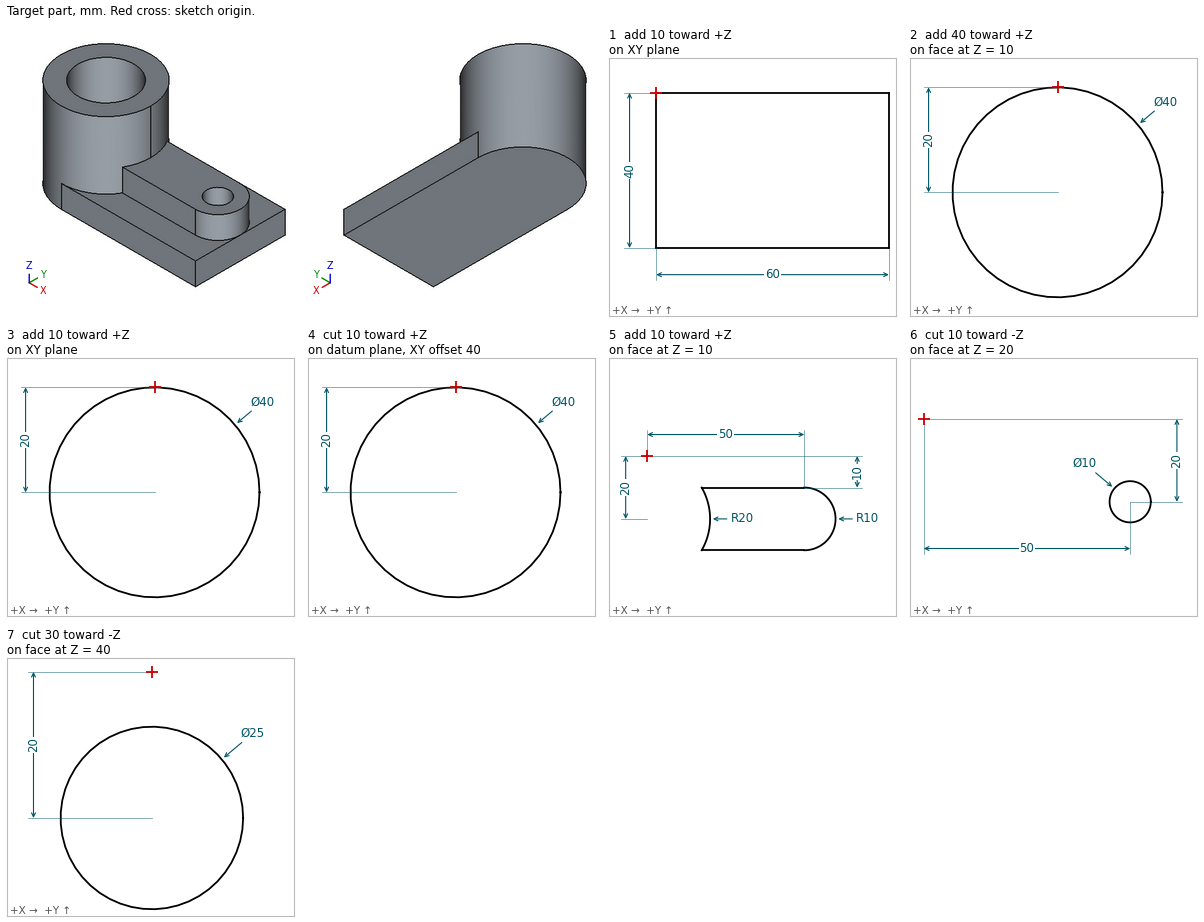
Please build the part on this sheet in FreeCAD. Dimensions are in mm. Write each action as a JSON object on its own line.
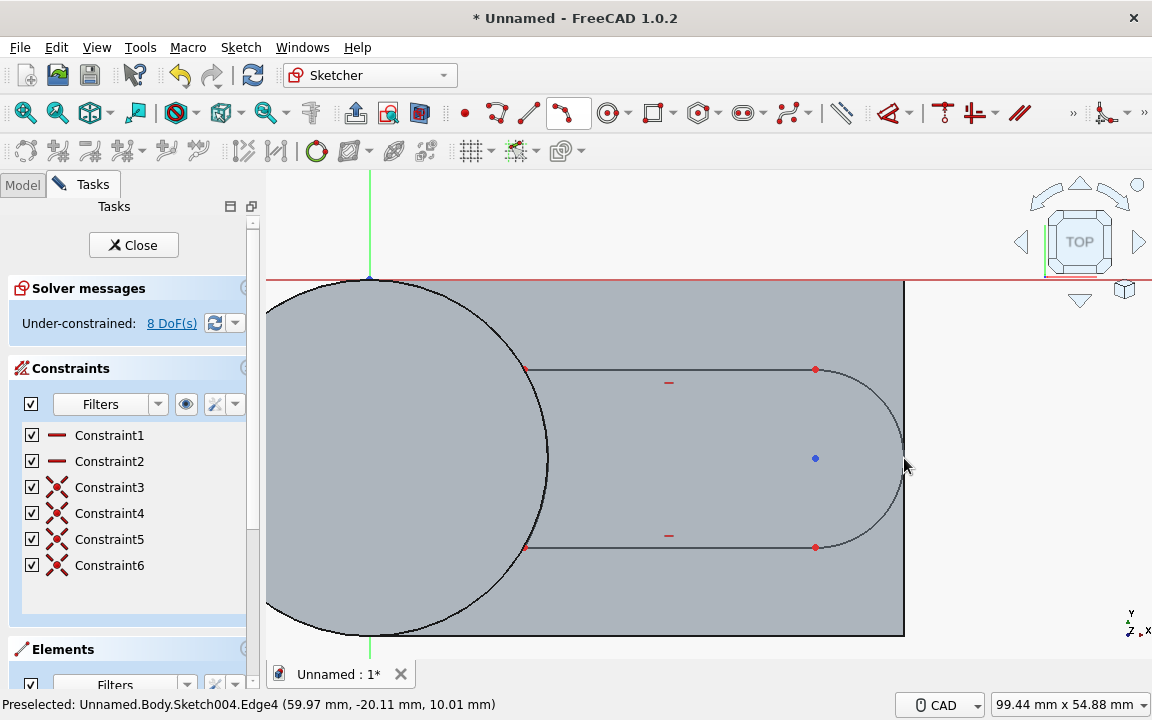
{"action": "left_click", "coordinate": [728, 370]}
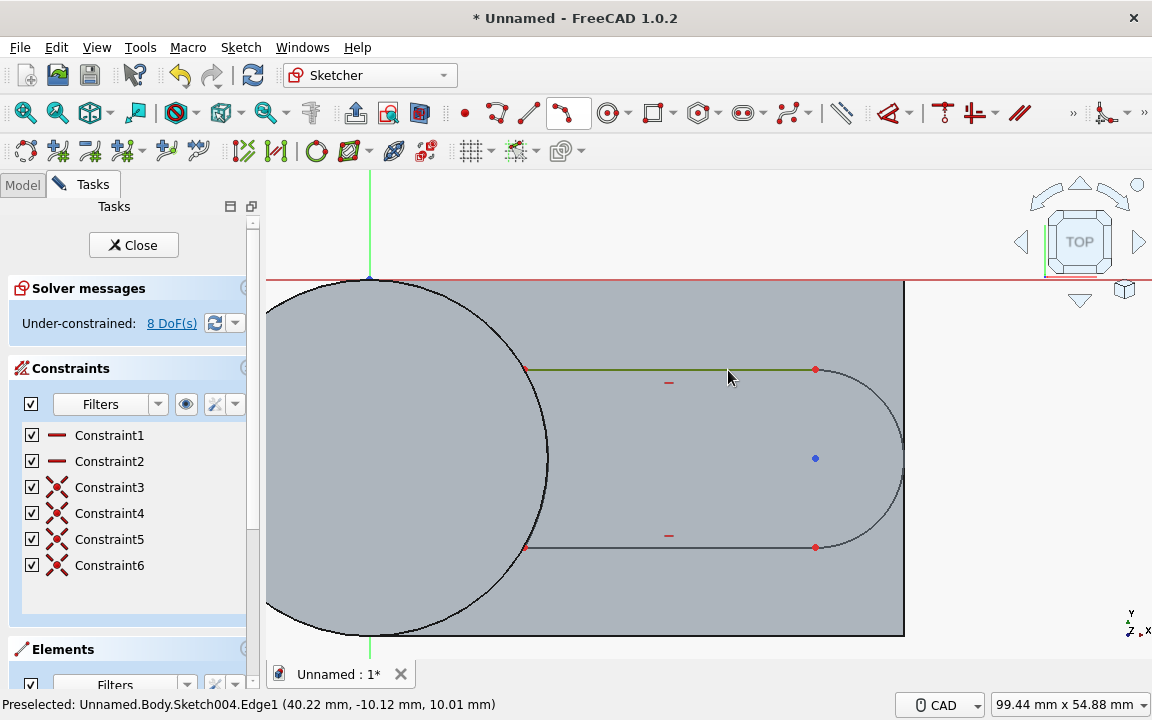
{"action": "left_click", "coordinate": [887, 511]}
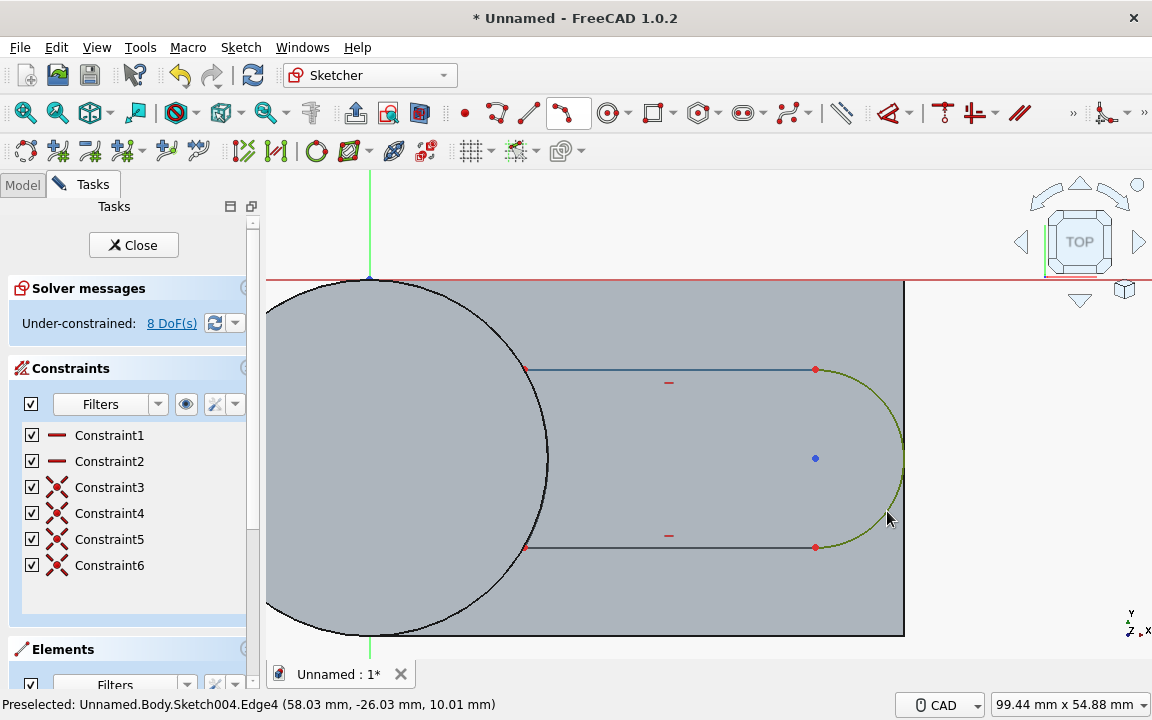
{"action": "key", "text": "t"}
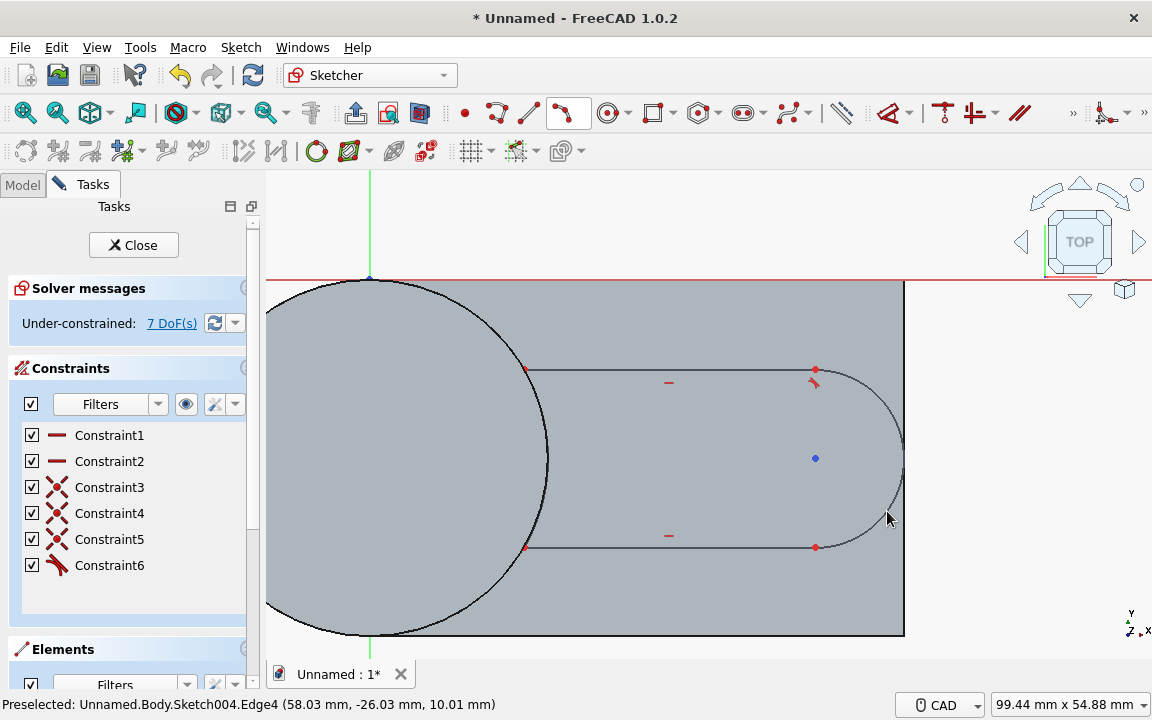
{"action": "left_click", "coordinate": [611, 548]}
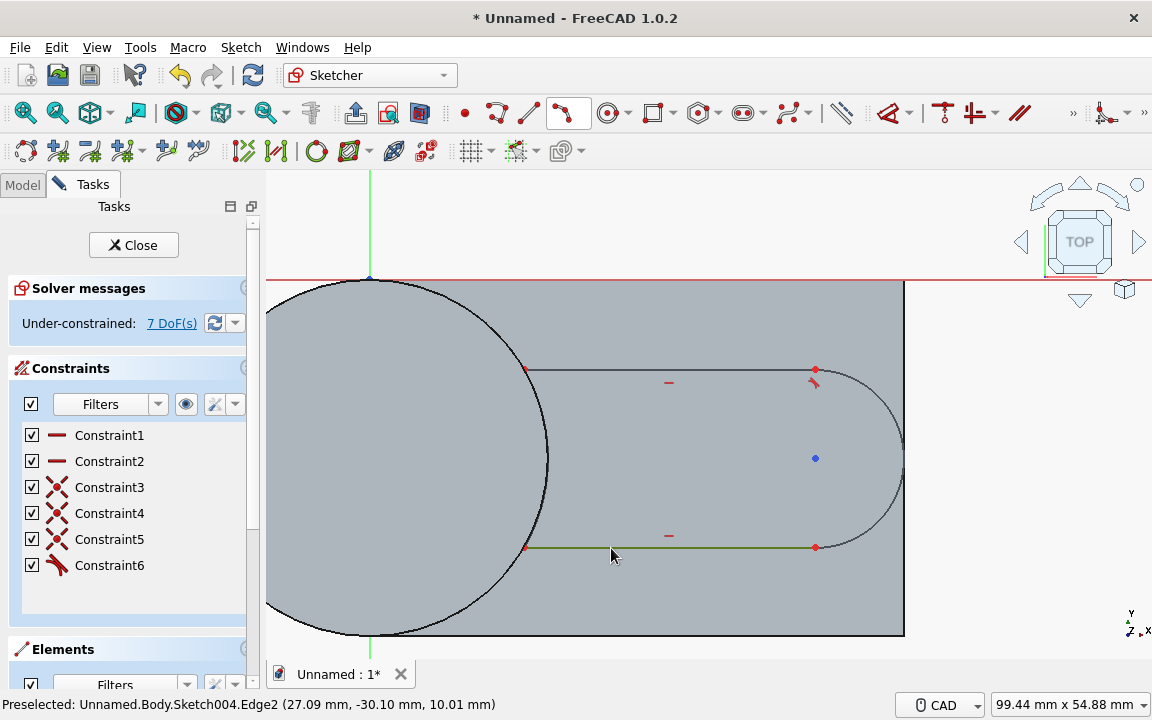
{"action": "left_click", "coordinate": [887, 511]}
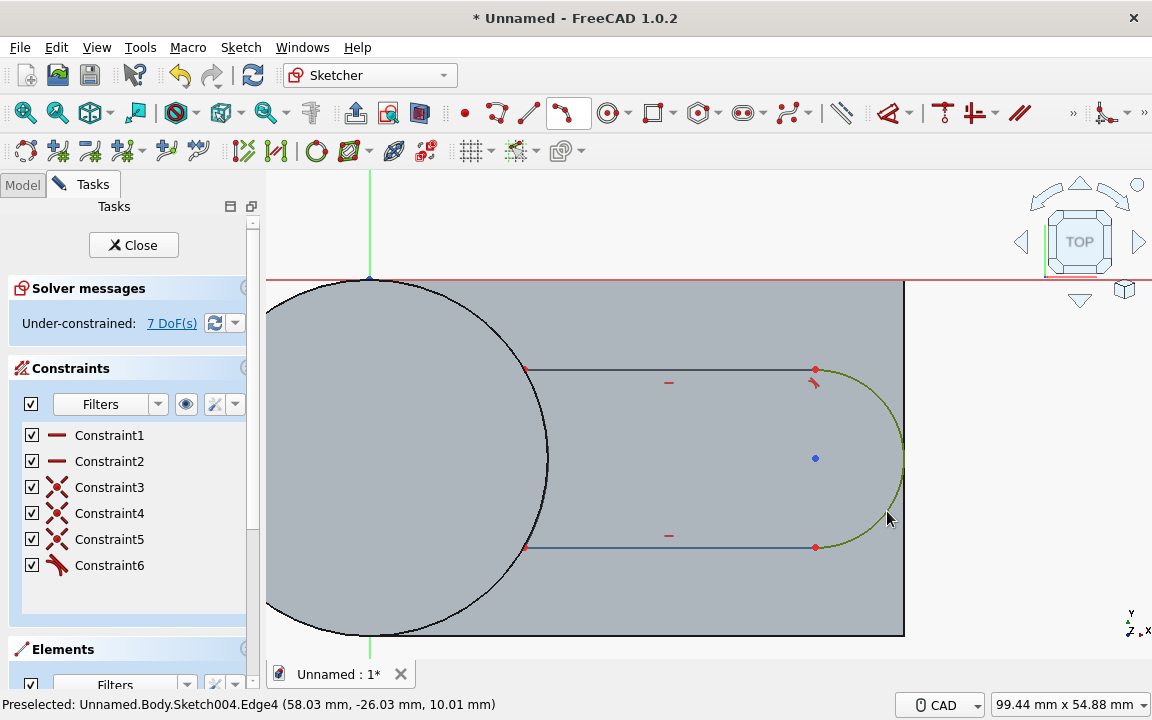
{"action": "key", "text": "t"}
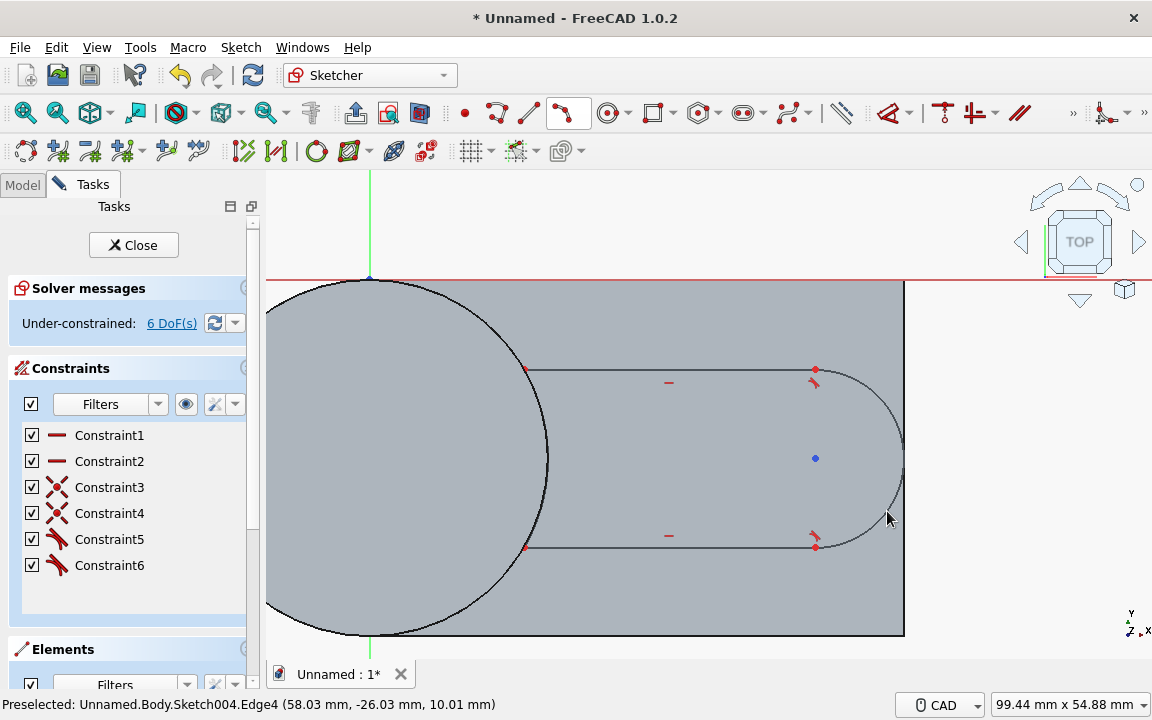
{"action": "left_click", "coordinate": [371, 459]}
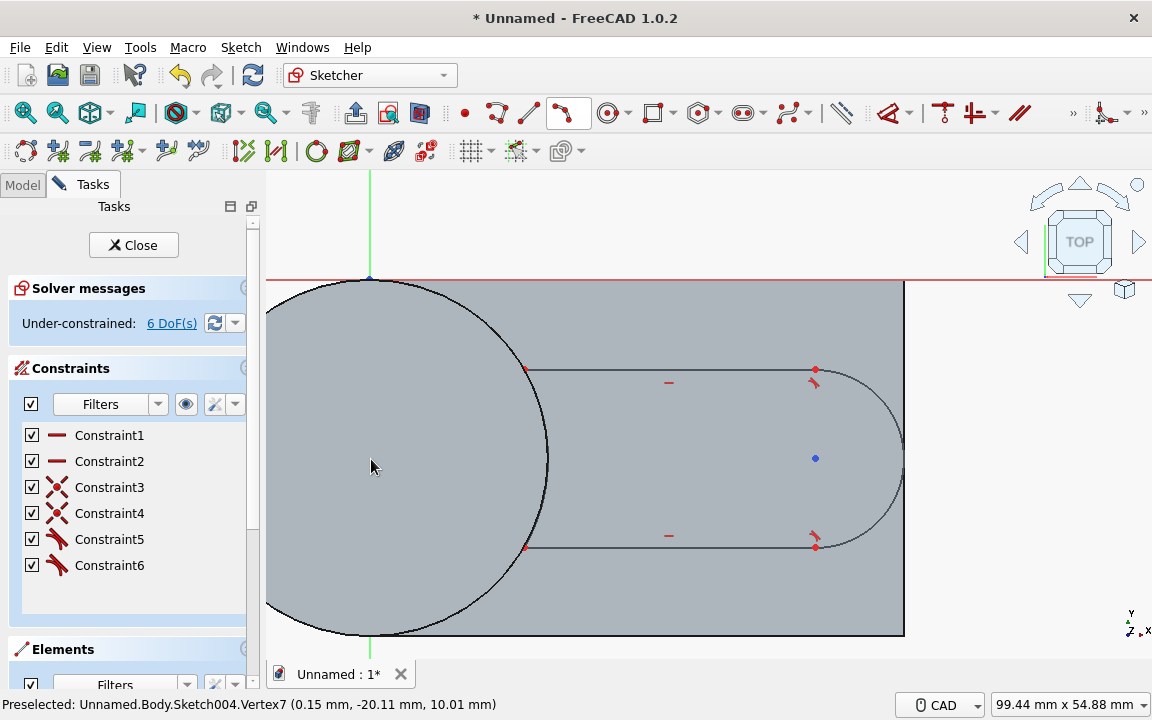
{"action": "left_click", "coordinate": [370, 600]}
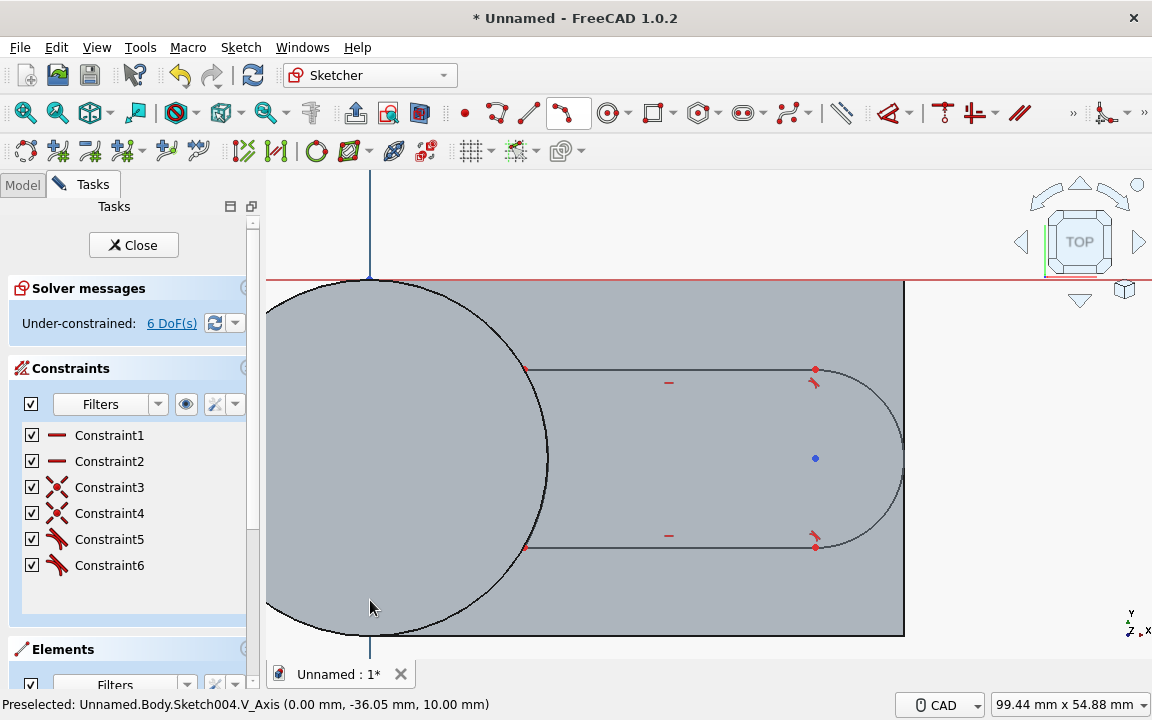
{"action": "left_click", "coordinate": [944, 114]}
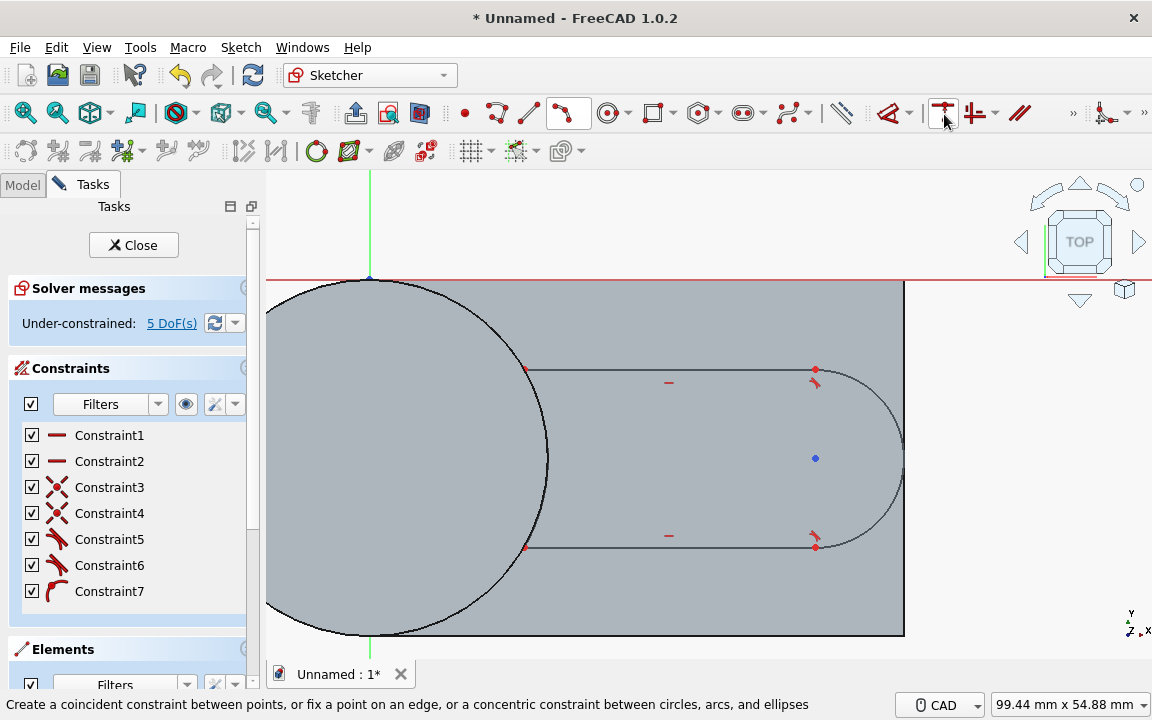
{"action": "left_click", "coordinate": [888, 114]}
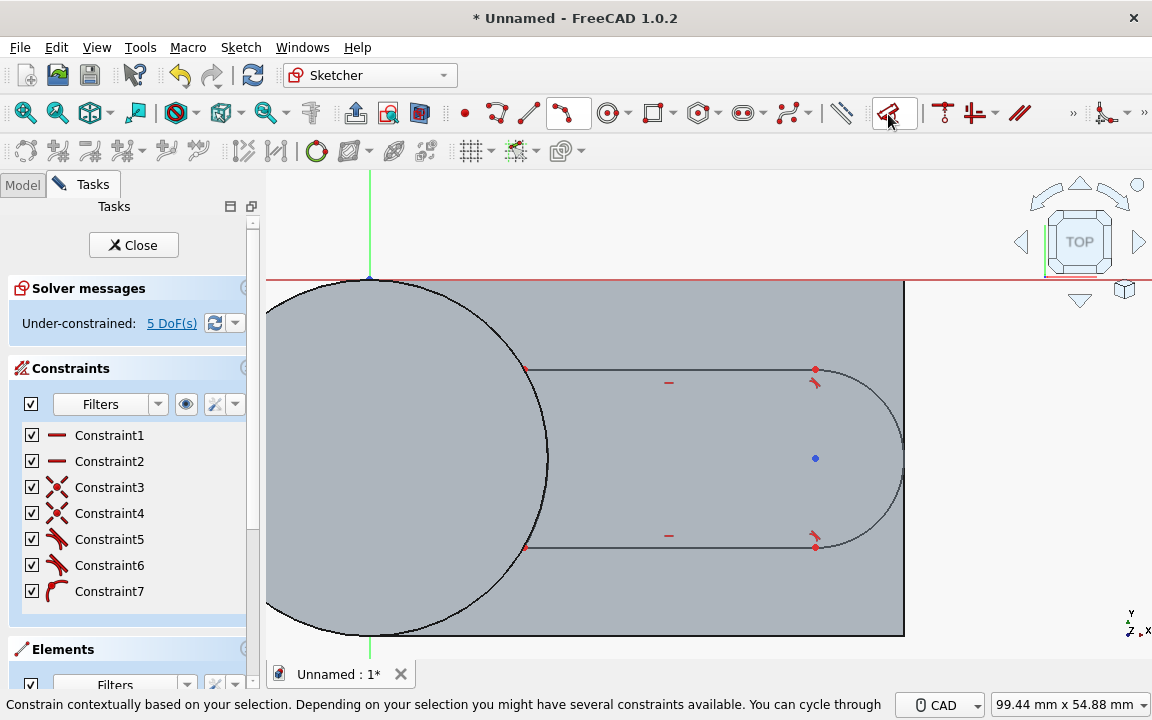
{"action": "left_click", "coordinate": [544, 496]}
{"action": "left_click", "coordinate": [575, 503]}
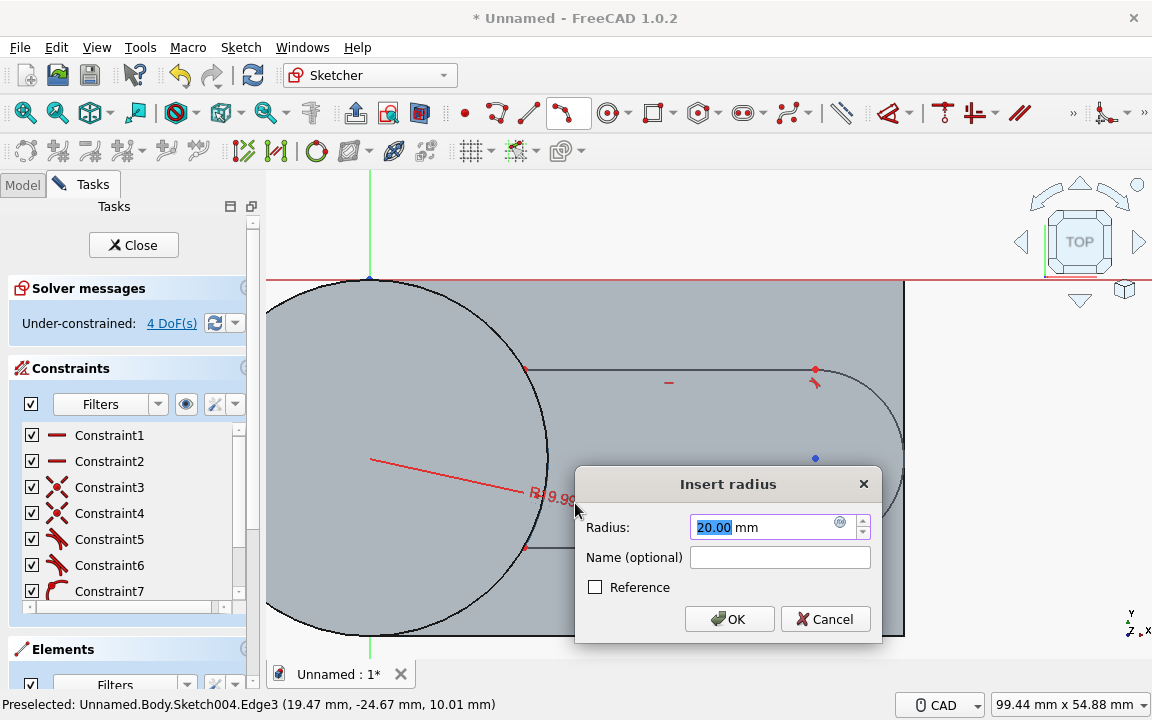
{"action": "type", "text": "20"}
{"action": "key", "text": "Return"}